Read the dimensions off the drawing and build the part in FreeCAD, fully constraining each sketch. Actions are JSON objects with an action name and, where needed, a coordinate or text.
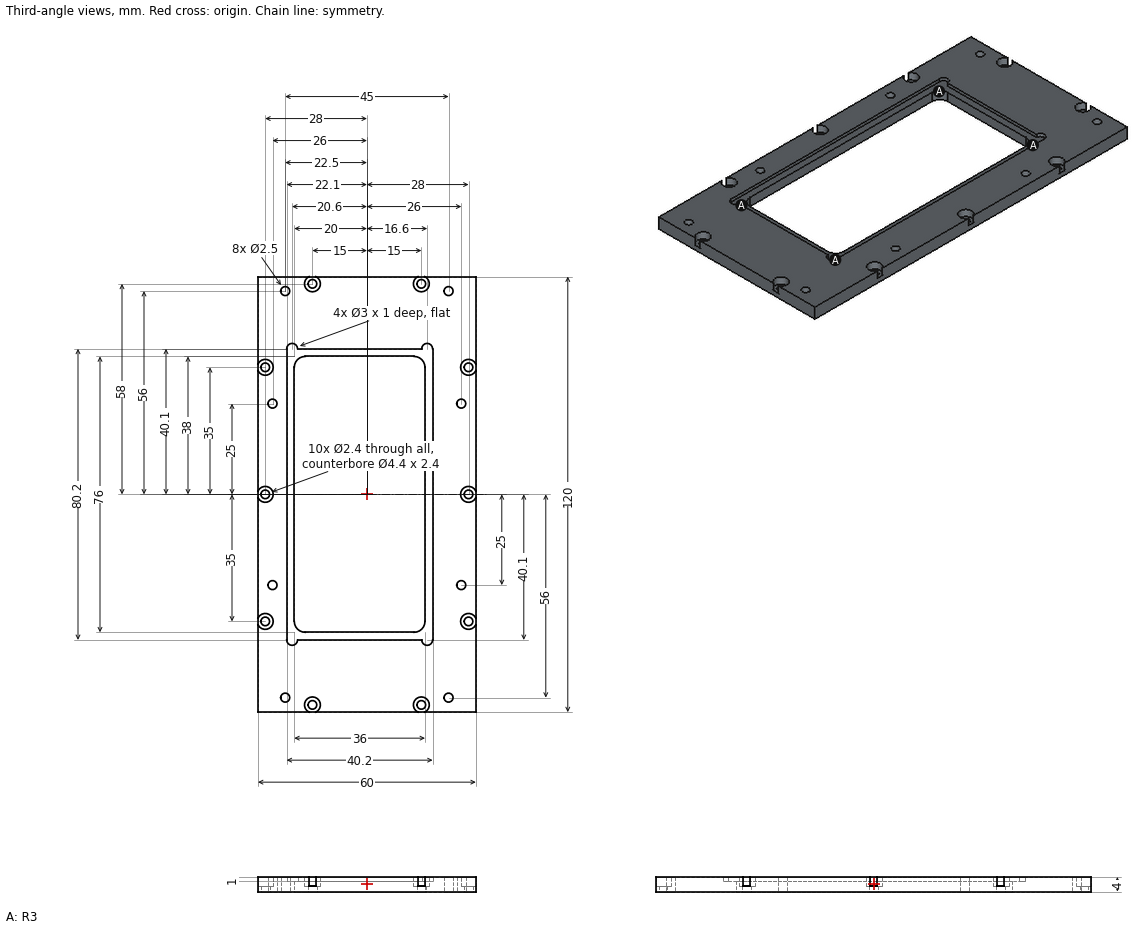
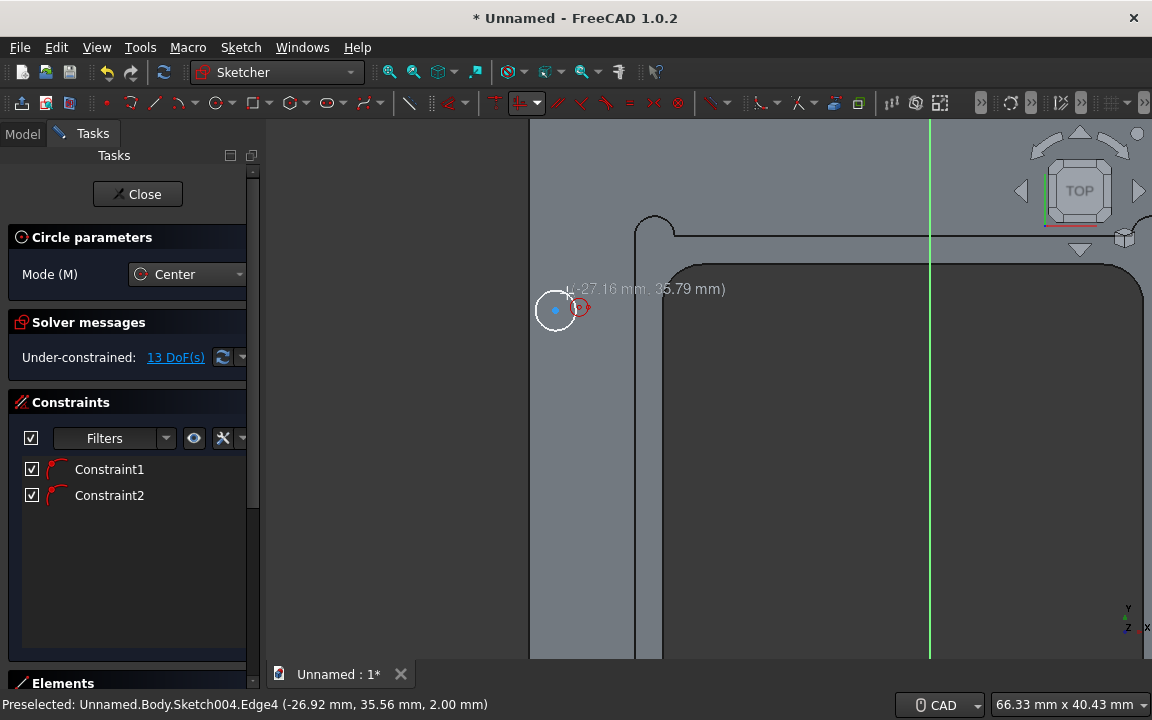
{"action": "scroll", "coordinate": [567, 292], "scroll_direction": "down", "scroll_amount": 8}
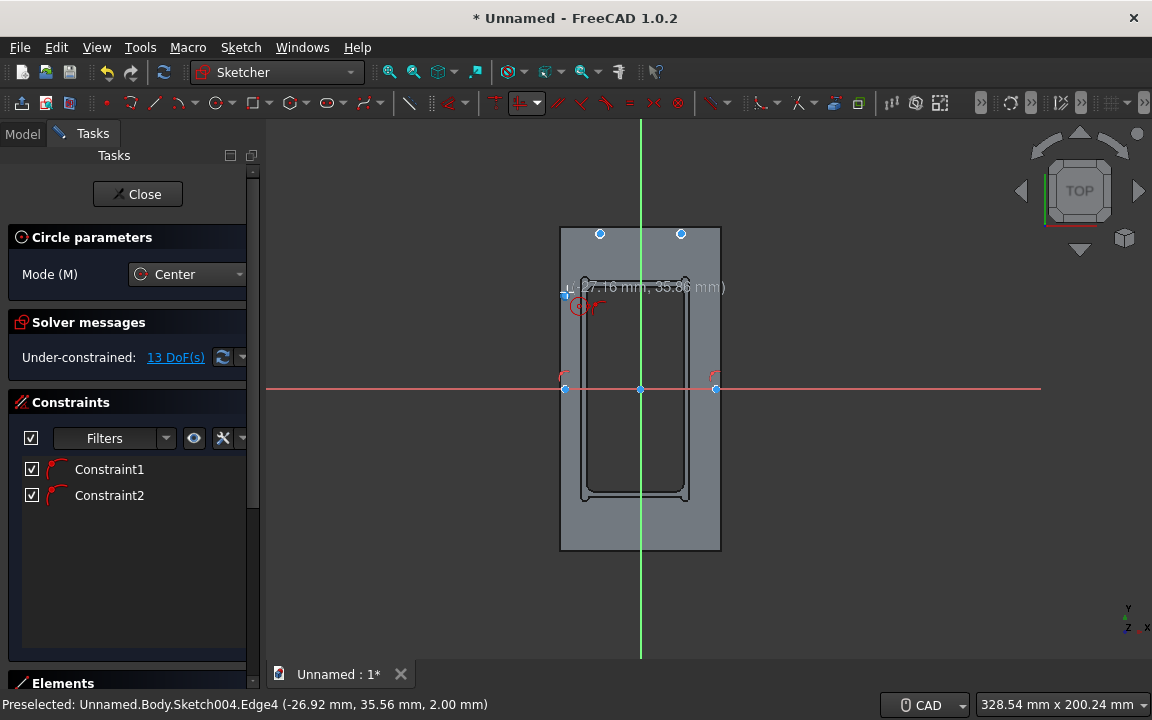
{"action": "scroll", "coordinate": [716, 295], "scroll_direction": "up", "scroll_amount": 10}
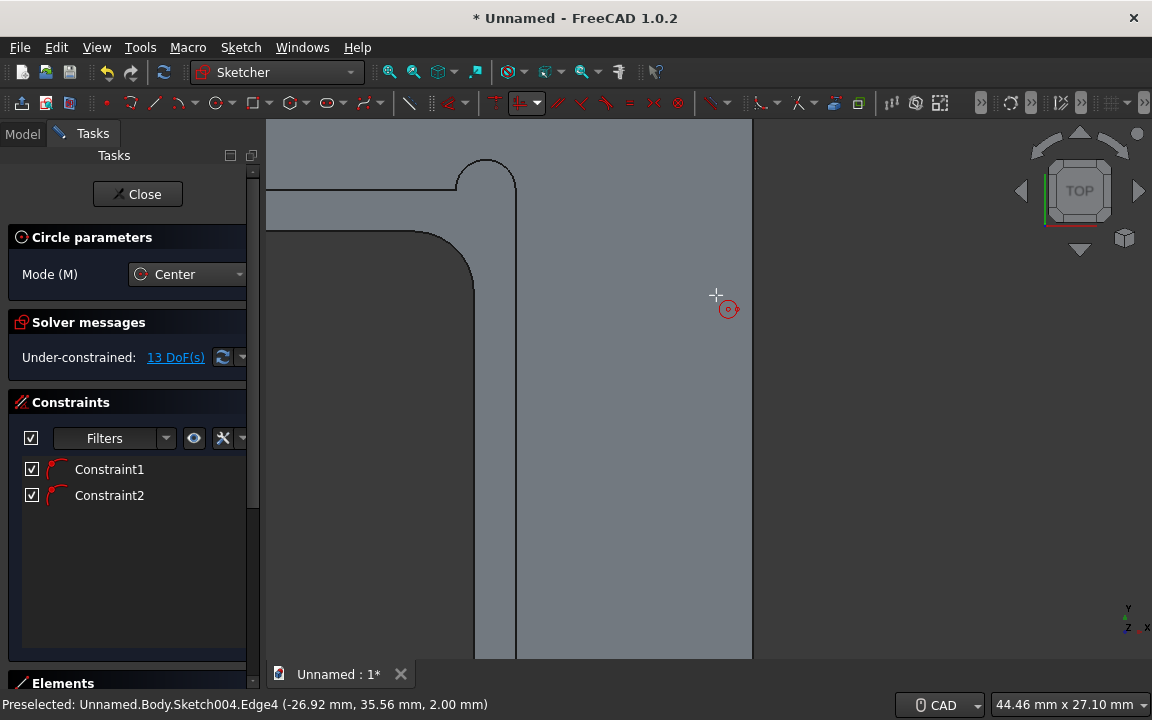
{"action": "scroll", "coordinate": [716, 295], "scroll_direction": "down", "scroll_amount": 10}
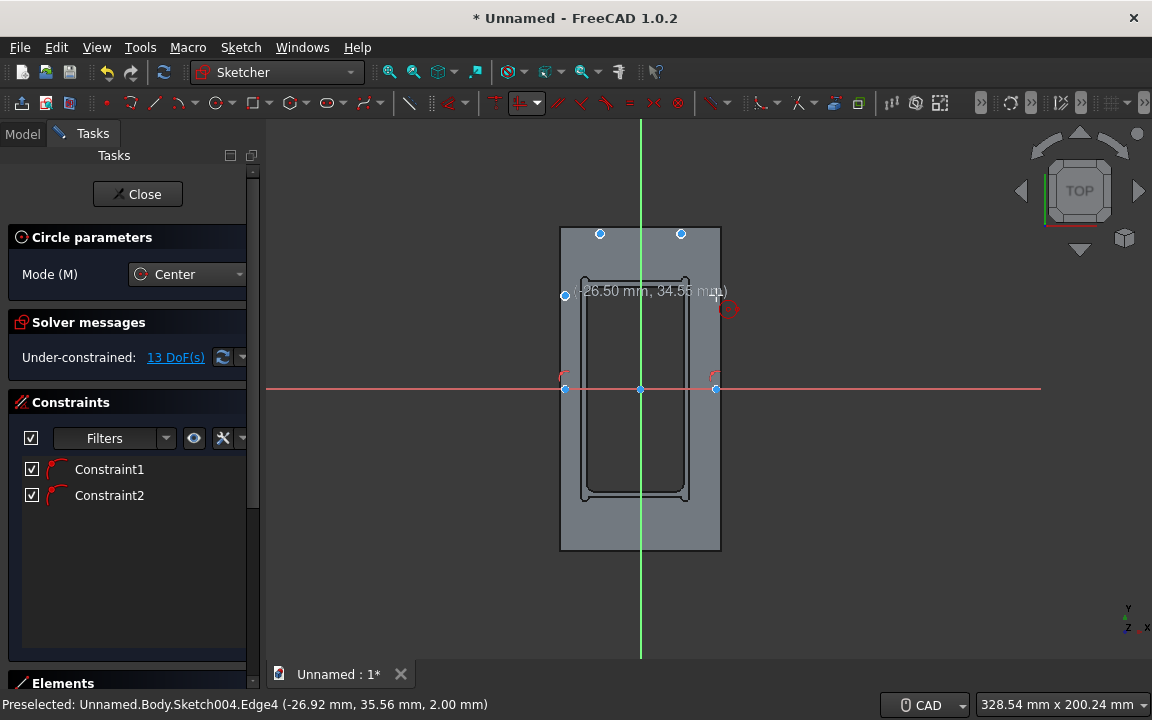
{"action": "left_click", "coordinate": [716, 295]}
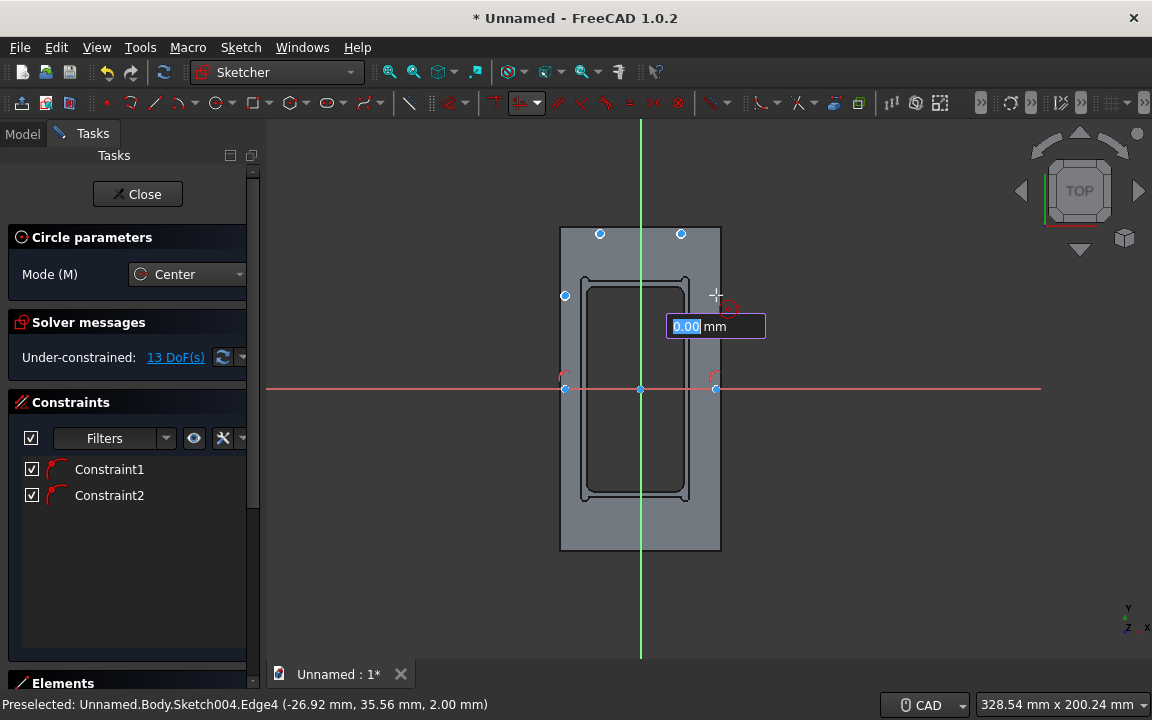
{"action": "scroll", "coordinate": [718, 292], "scroll_direction": "up", "scroll_amount": 8}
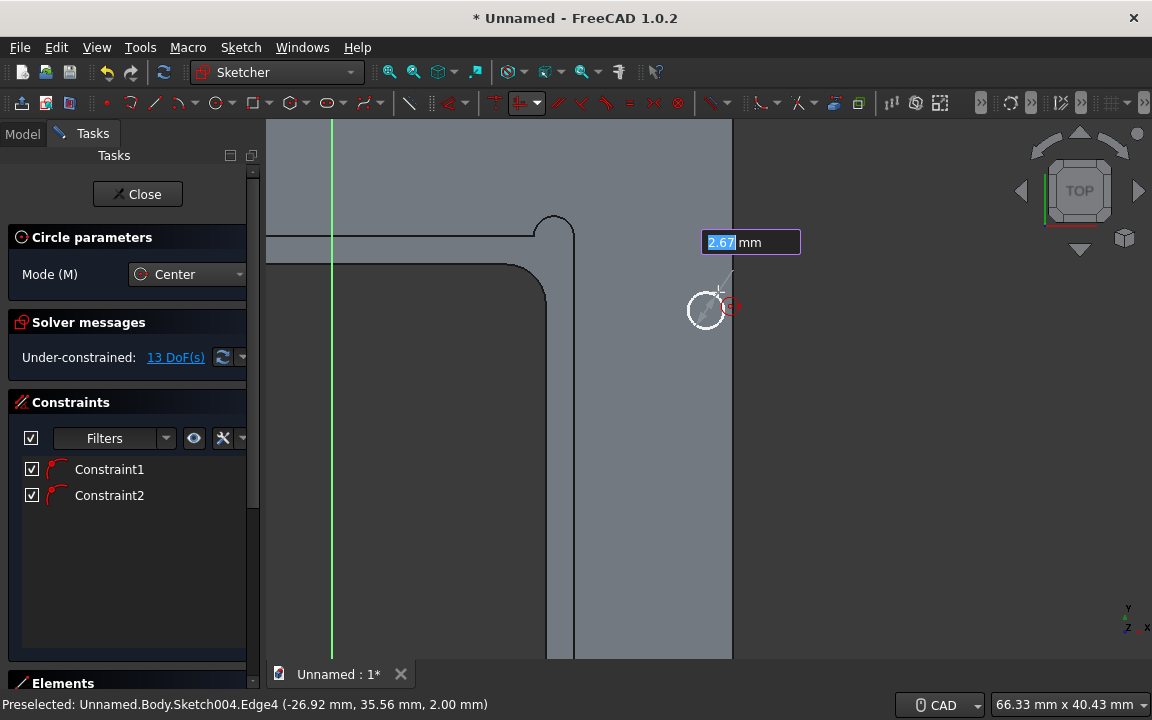
{"action": "left_click", "coordinate": [718, 293]}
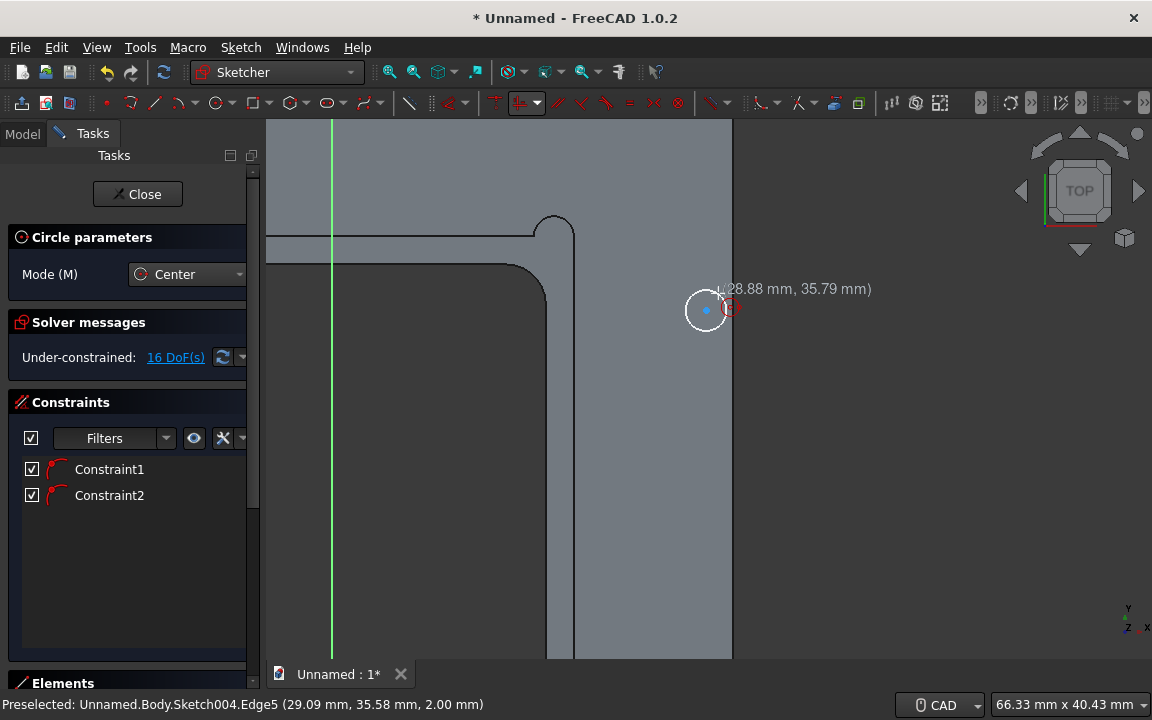
{"action": "scroll", "coordinate": [718, 292], "scroll_direction": "down", "scroll_amount": 8}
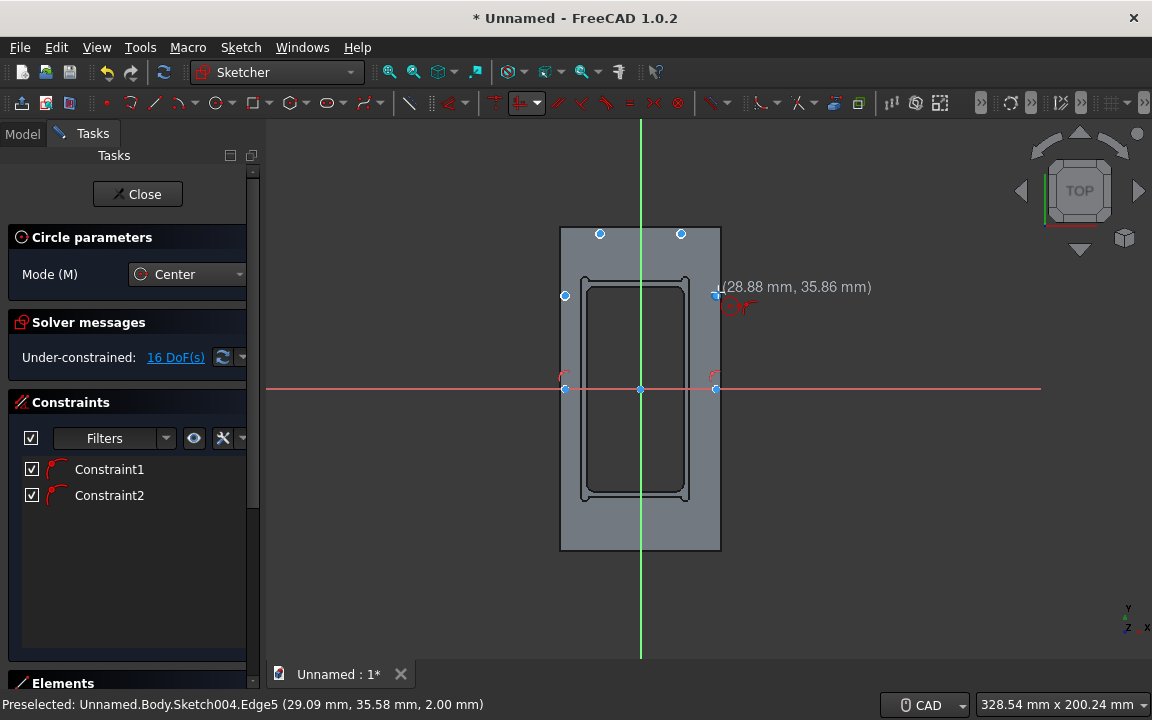
{"action": "scroll", "coordinate": [565, 484], "scroll_direction": "up", "scroll_amount": 10}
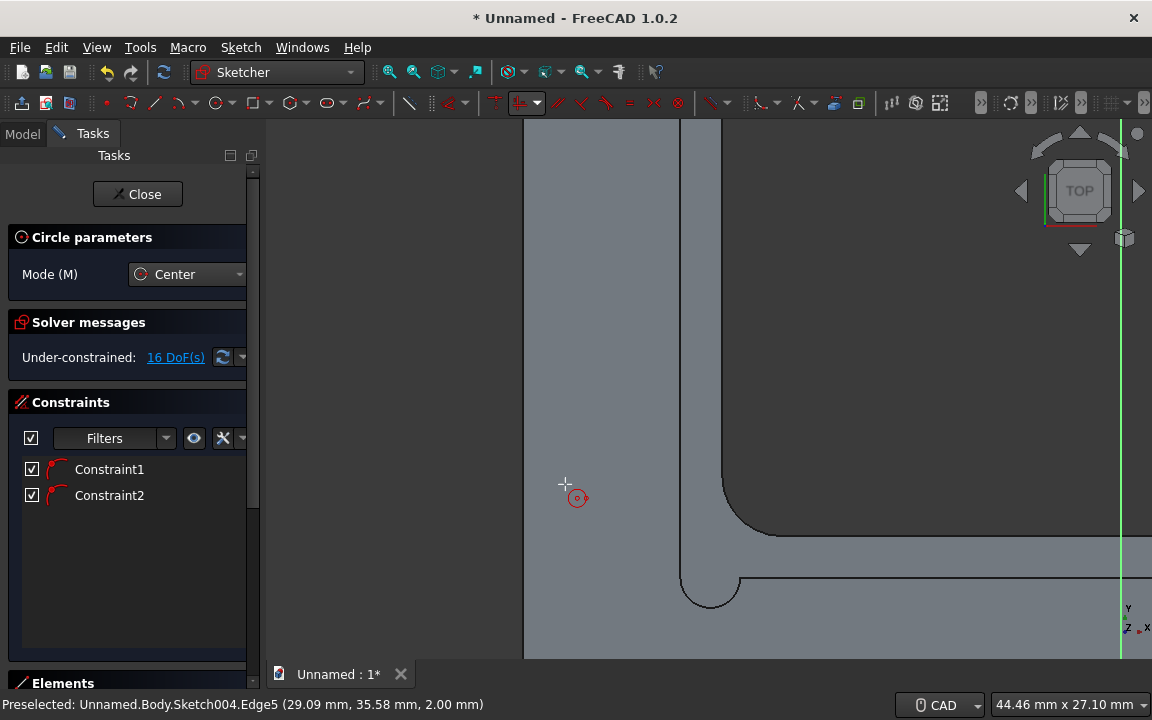
{"action": "scroll", "coordinate": [565, 484], "scroll_direction": "down", "scroll_amount": 10}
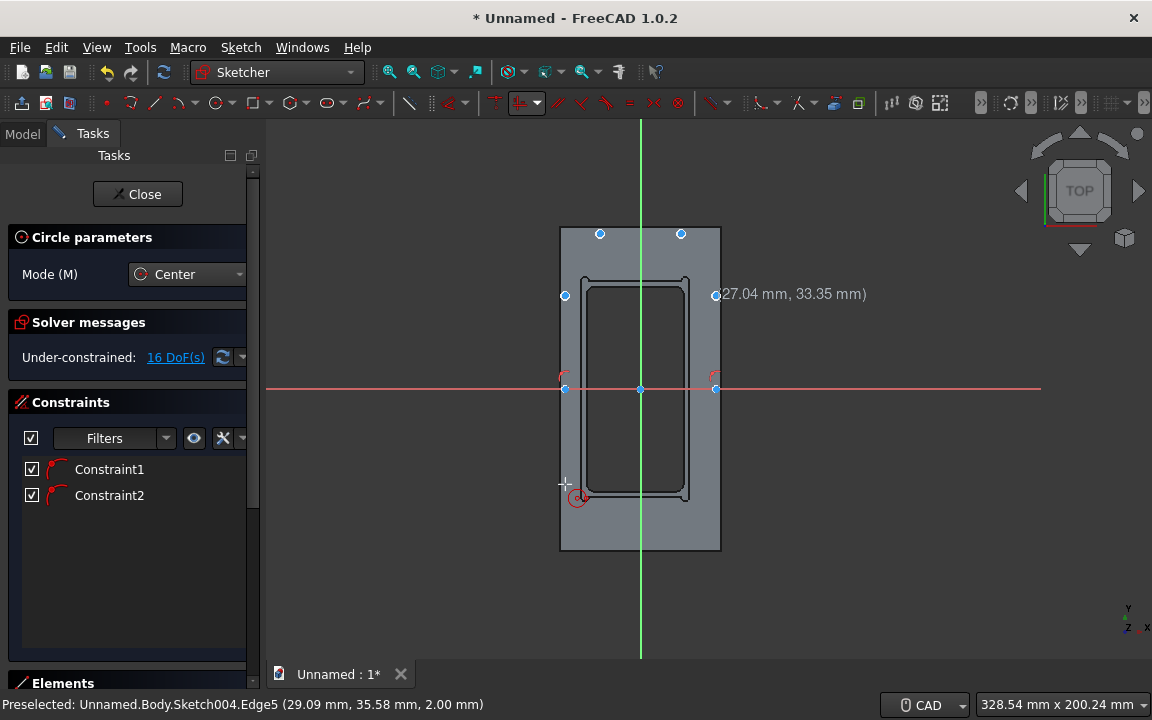
{"action": "left_click", "coordinate": [565, 484]}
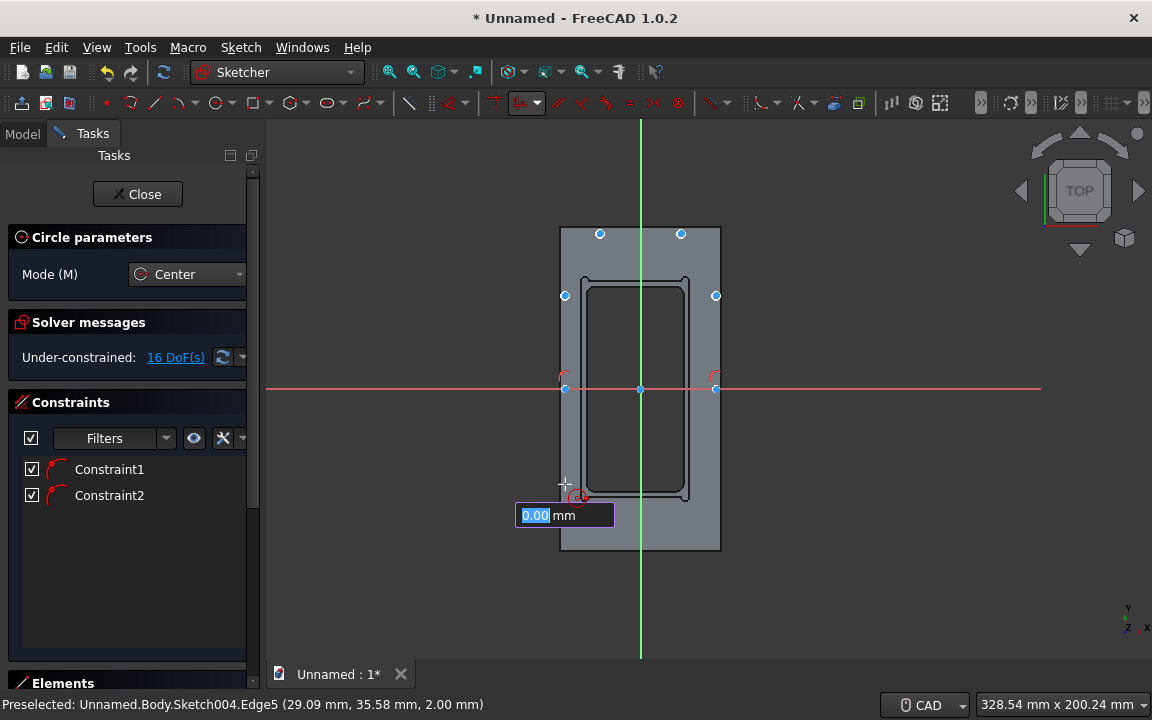
{"action": "scroll", "coordinate": [567, 481], "scroll_direction": "up", "scroll_amount": 8}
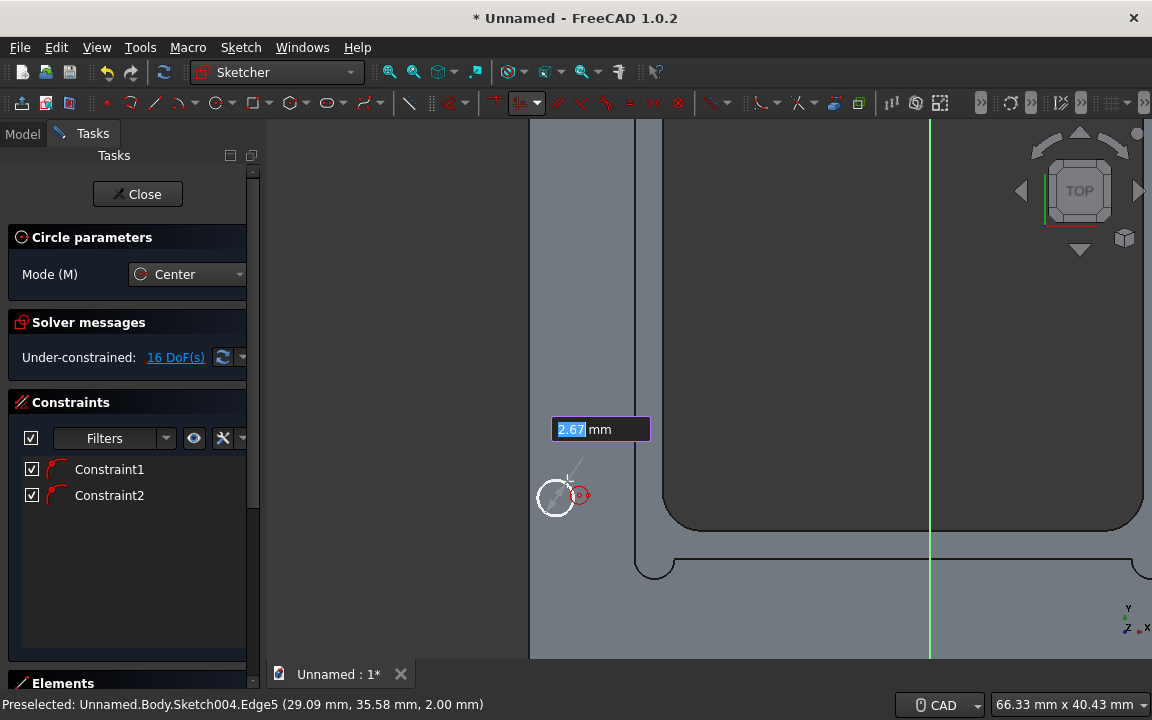
{"action": "left_click", "coordinate": [567, 480]}